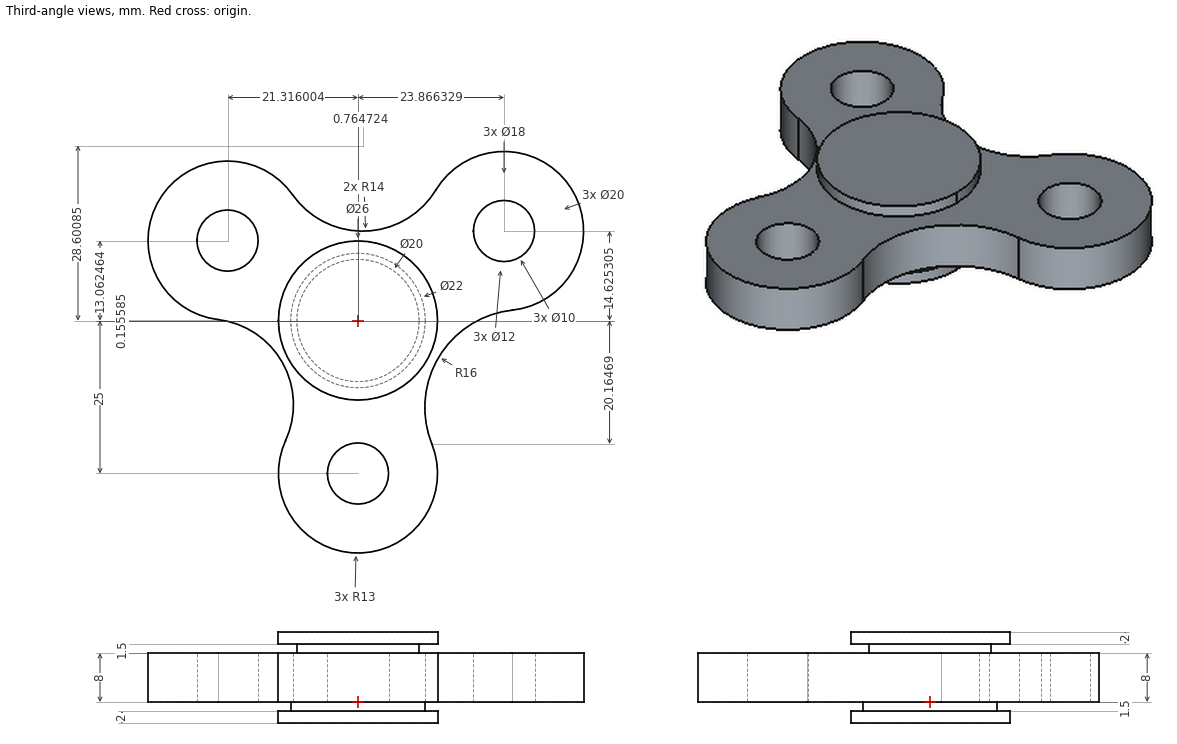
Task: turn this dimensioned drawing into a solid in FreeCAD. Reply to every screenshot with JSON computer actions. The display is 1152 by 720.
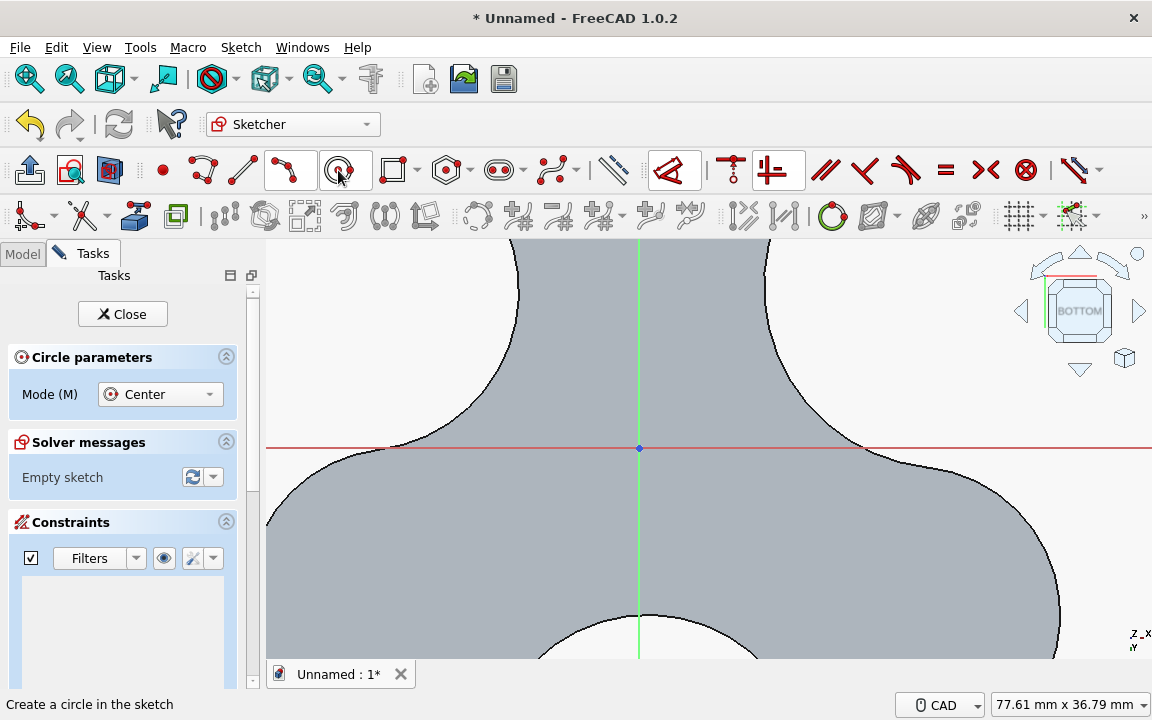
{"action": "left_click", "coordinate": [639, 448]}
{"action": "mouse_move", "coordinate": [728, 359]}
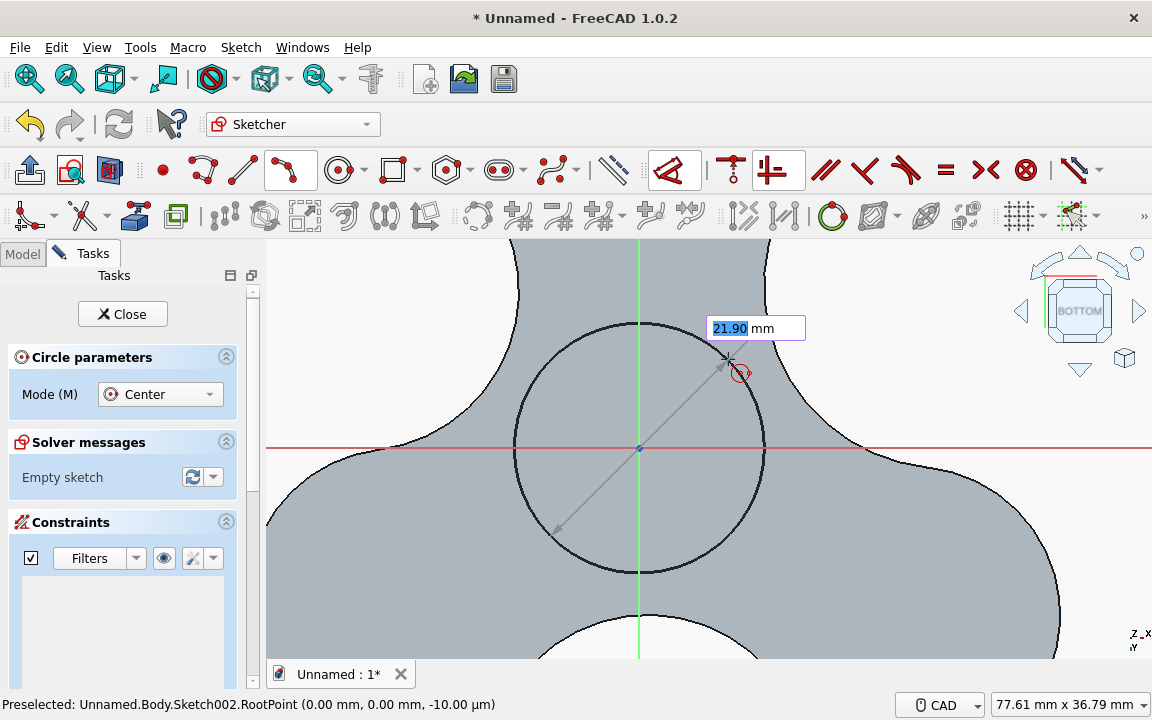
{"action": "type", "text": "22"}
{"action": "key", "text": "Return"}
{"action": "key", "text": "Escape"}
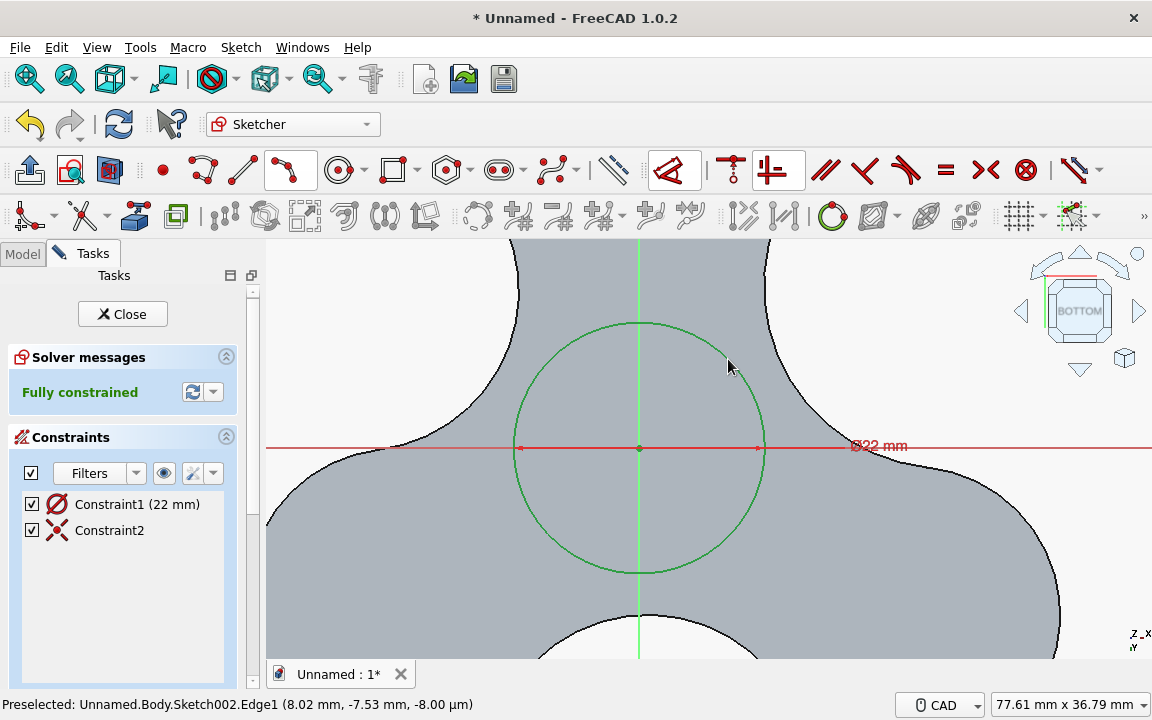
{"action": "left_click", "coordinate": [123, 314]}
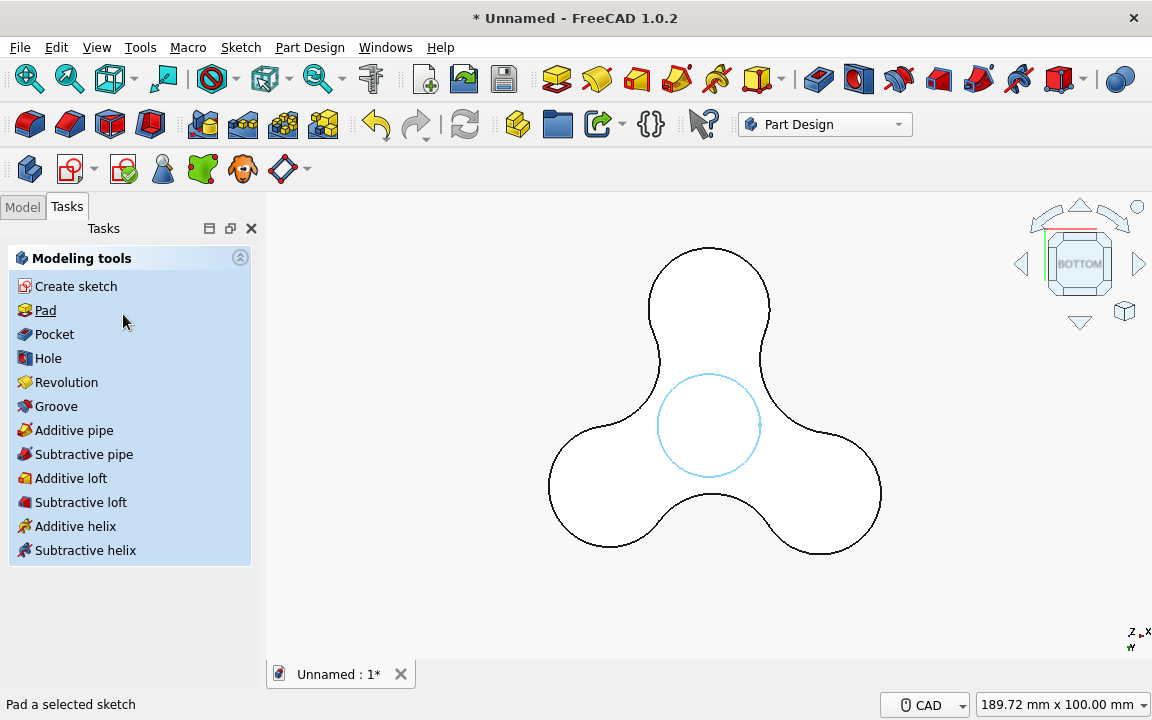
{"action": "left_click", "coordinate": [558, 80]}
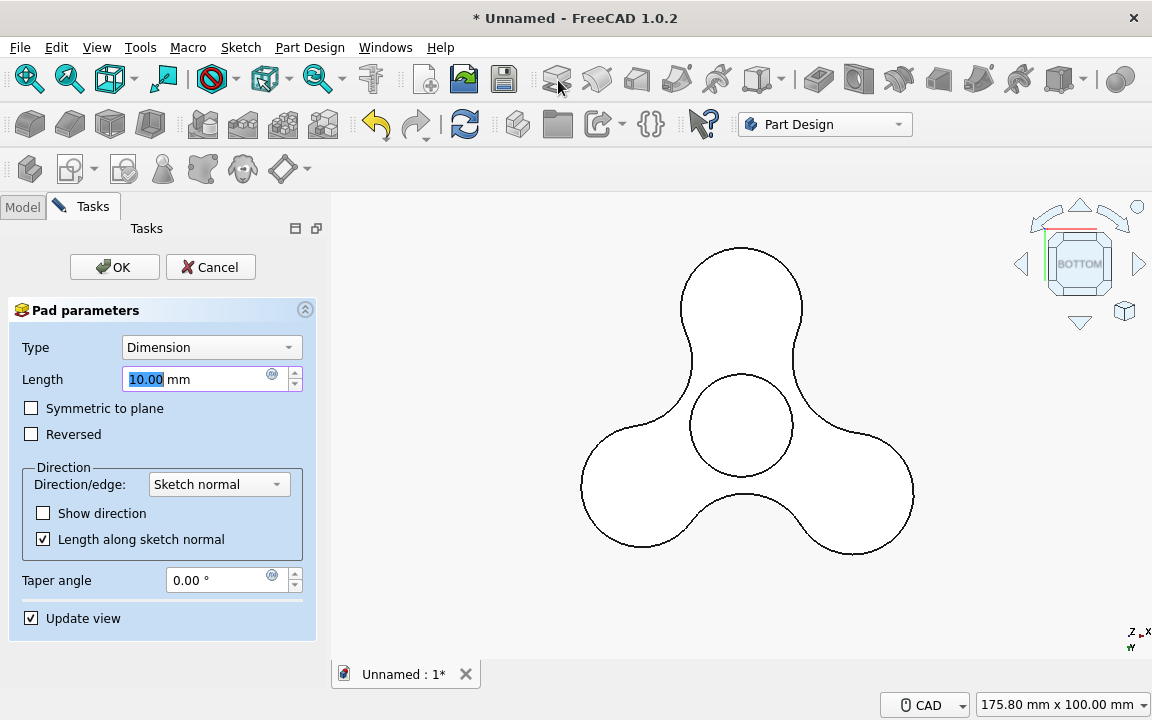
{"action": "type", "text": "1.5"}
{"action": "key", "text": "Tab"}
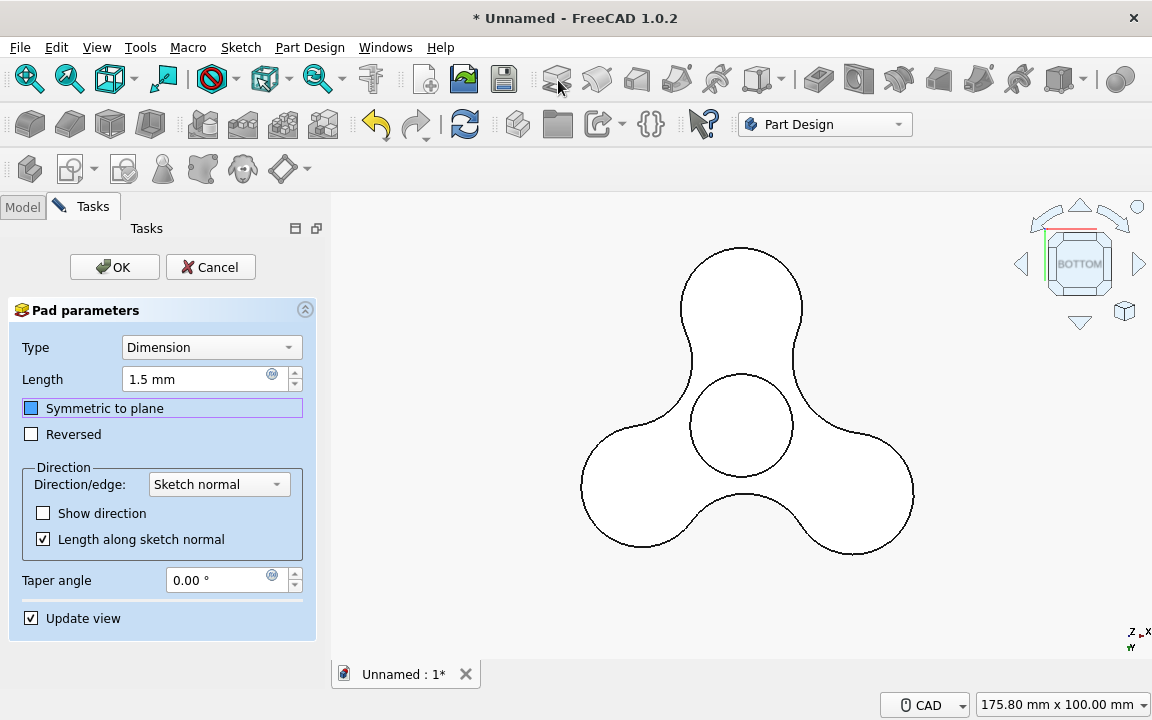
{"action": "left_click", "coordinate": [115, 267]}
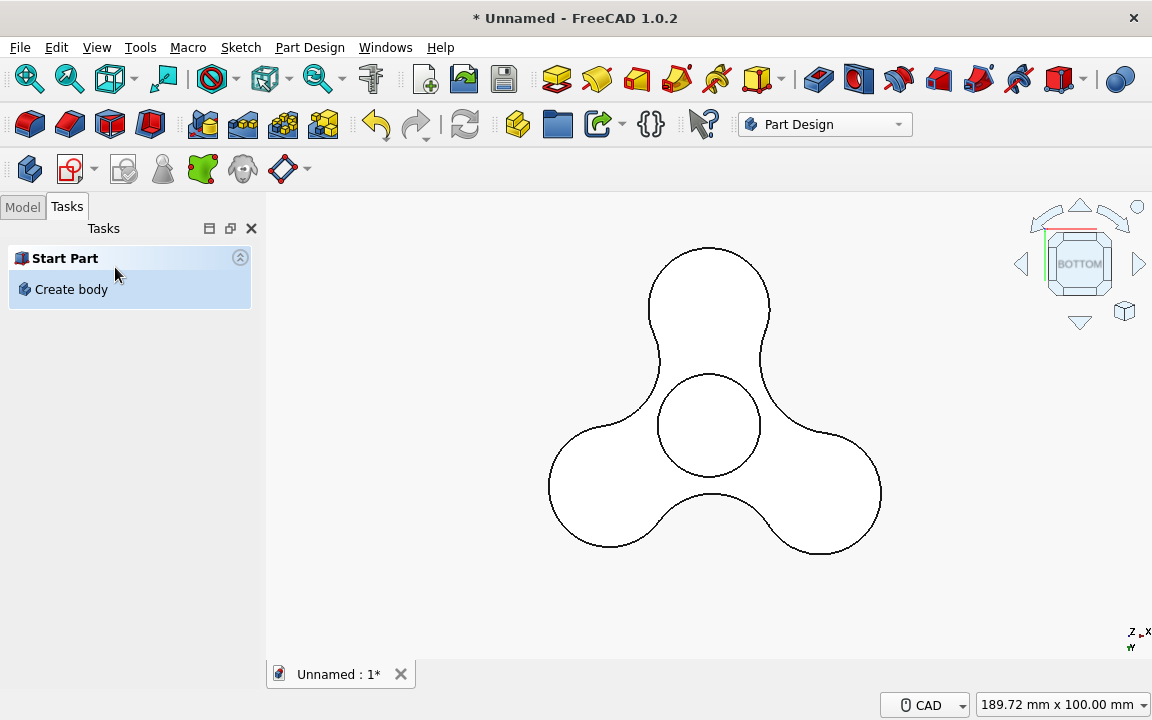
{"action": "left_click", "coordinate": [709, 425]}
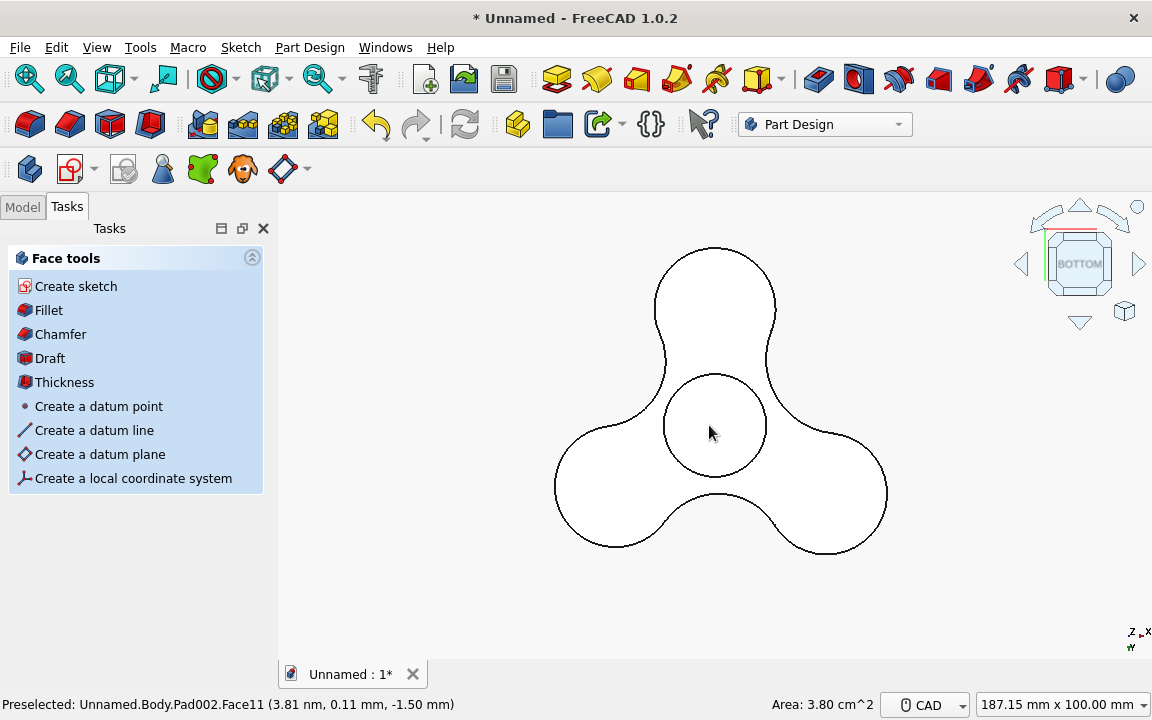
{"action": "left_click", "coordinate": [70, 170]}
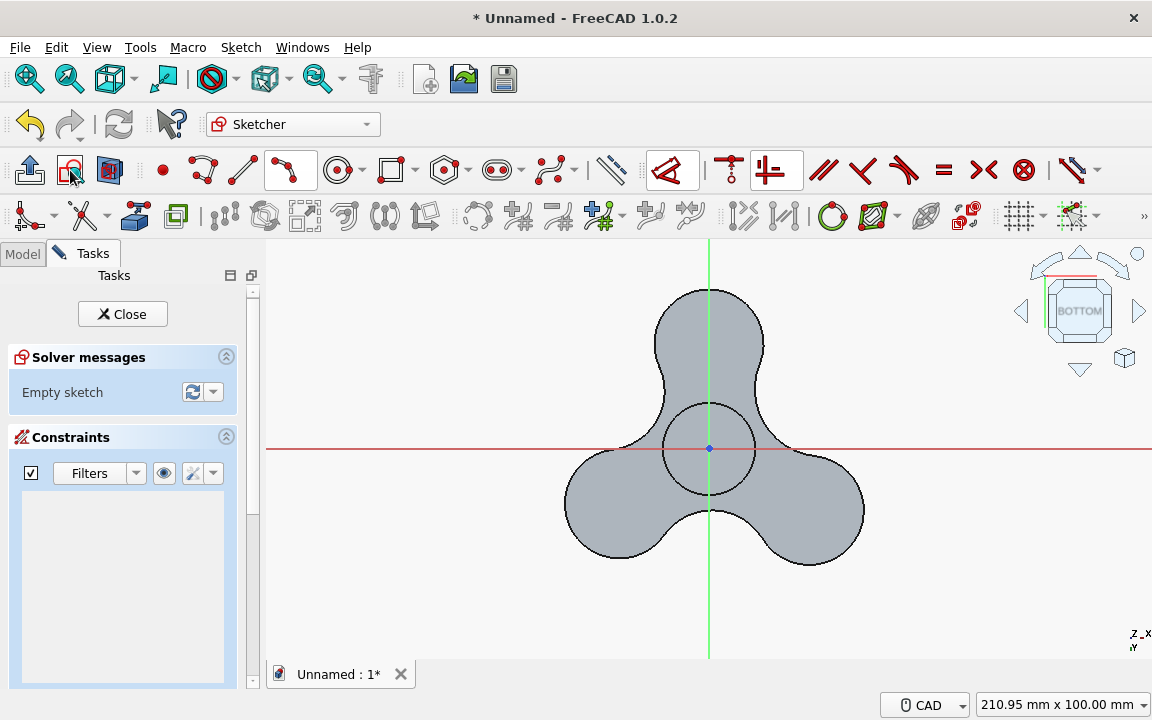
{"action": "scroll", "coordinate": [765, 449], "scroll_direction": "up", "scroll_amount": 4}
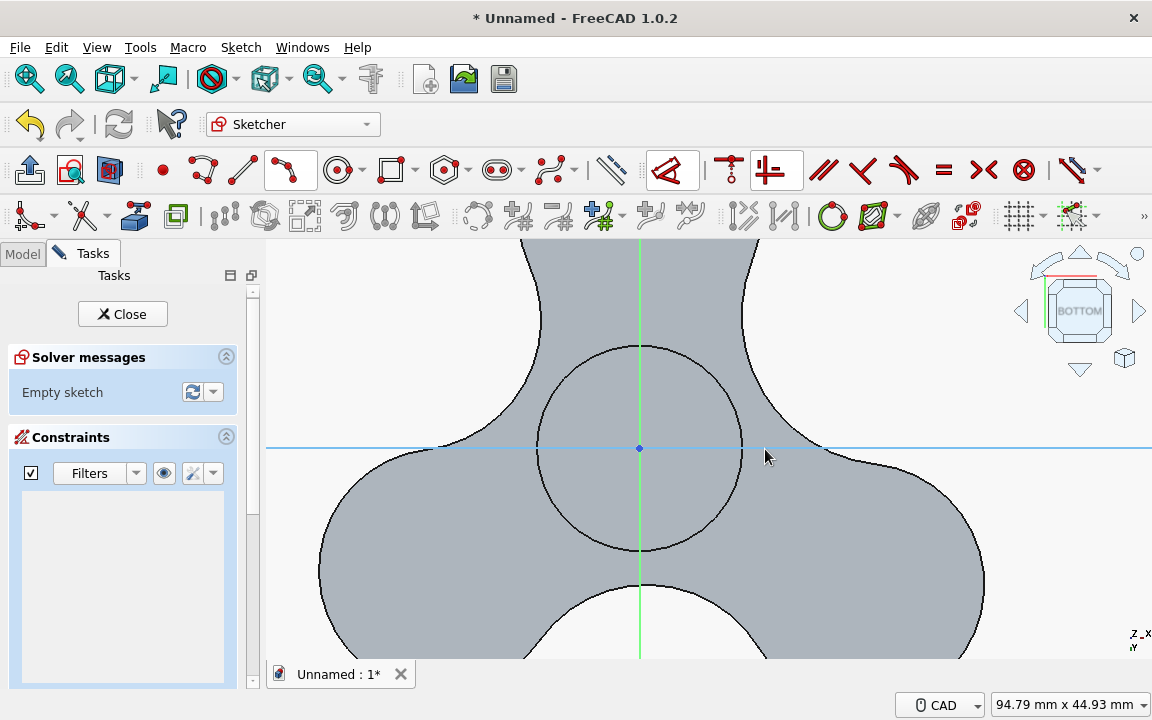
{"action": "left_click", "coordinate": [338, 170]}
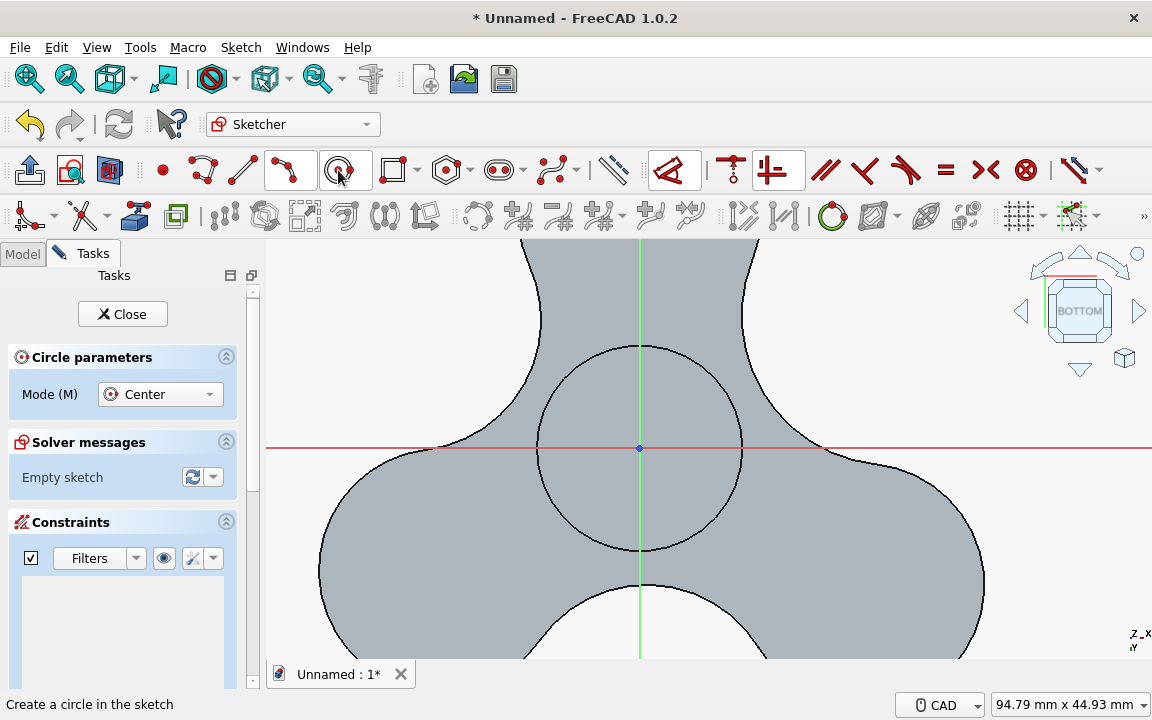
{"action": "left_click", "coordinate": [640, 448]}
{"action": "mouse_move", "coordinate": [726, 362]}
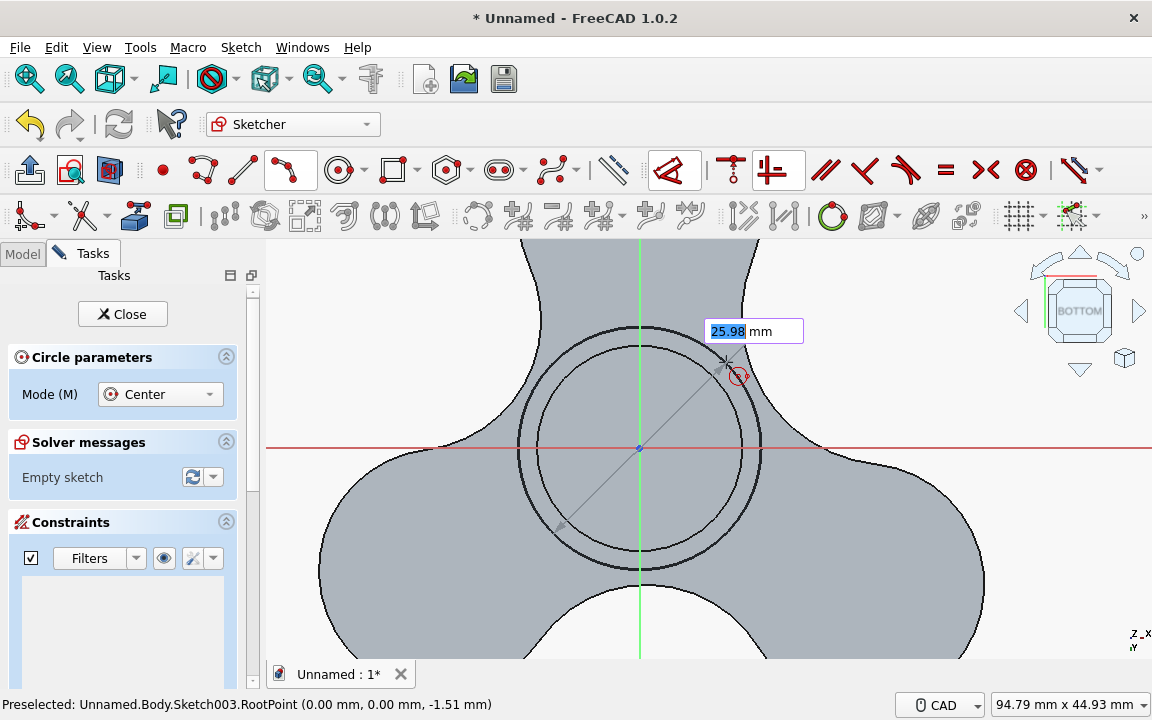
{"action": "type", "text": "26"}
{"action": "key", "text": "Return"}
{"action": "key", "text": "Escape"}